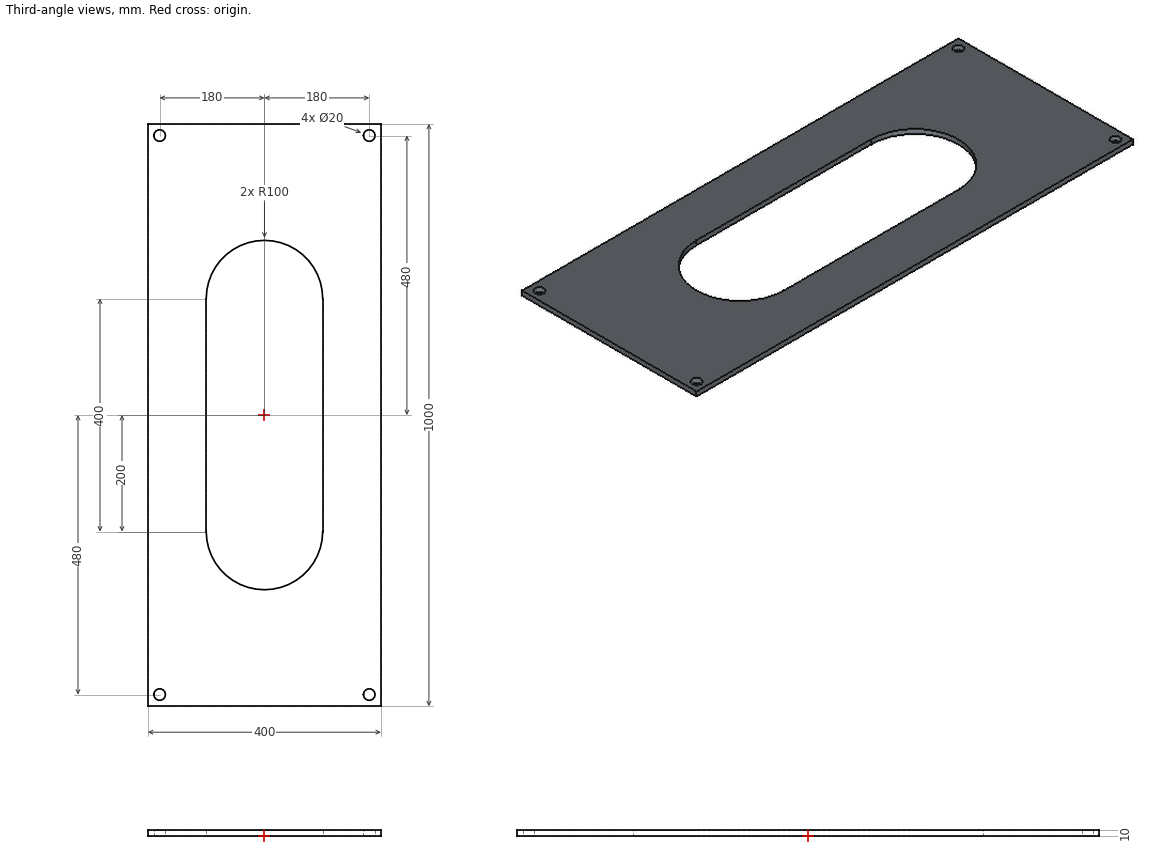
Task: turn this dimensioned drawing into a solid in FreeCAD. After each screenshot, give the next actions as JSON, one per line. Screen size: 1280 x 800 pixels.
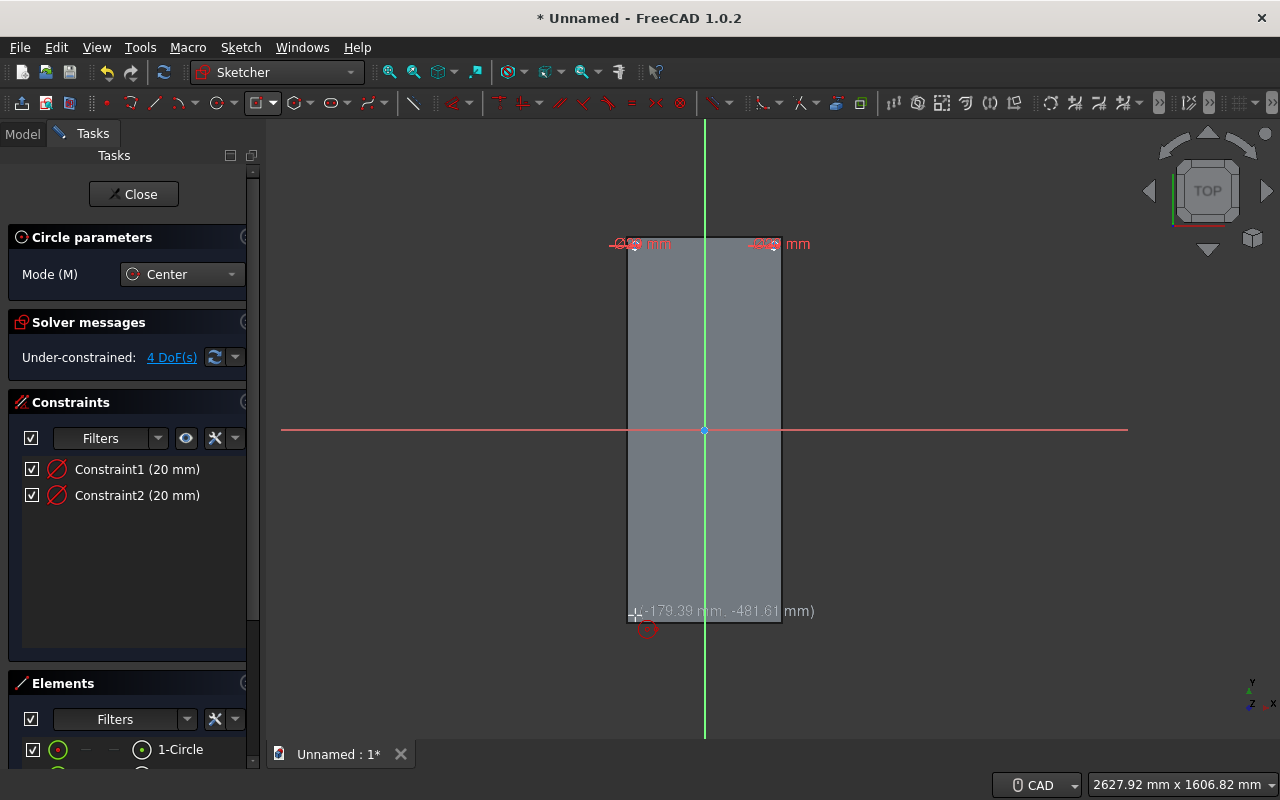
{"action": "left_click", "coordinate": [635, 615]}
{"action": "mouse_move", "coordinate": [638, 612]}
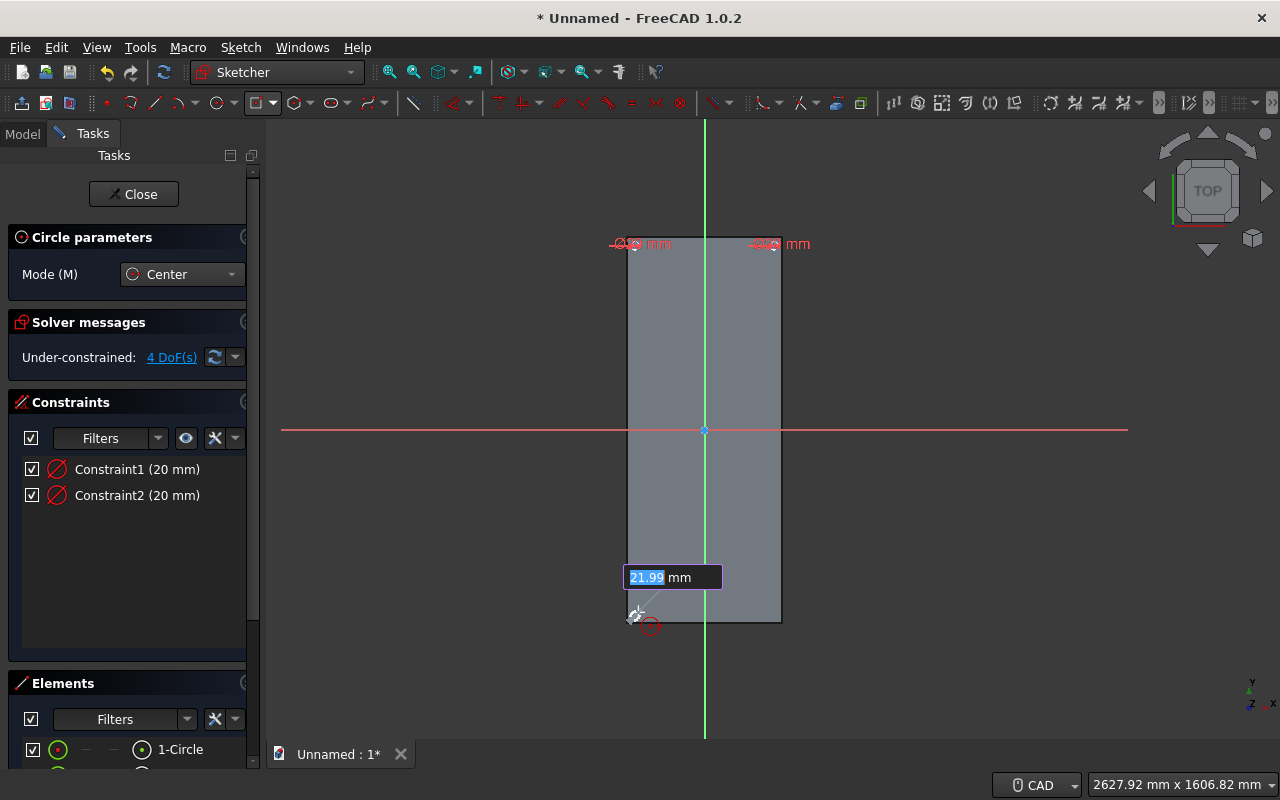
{"action": "type", "text": "20"}
{"action": "key", "text": "Return"}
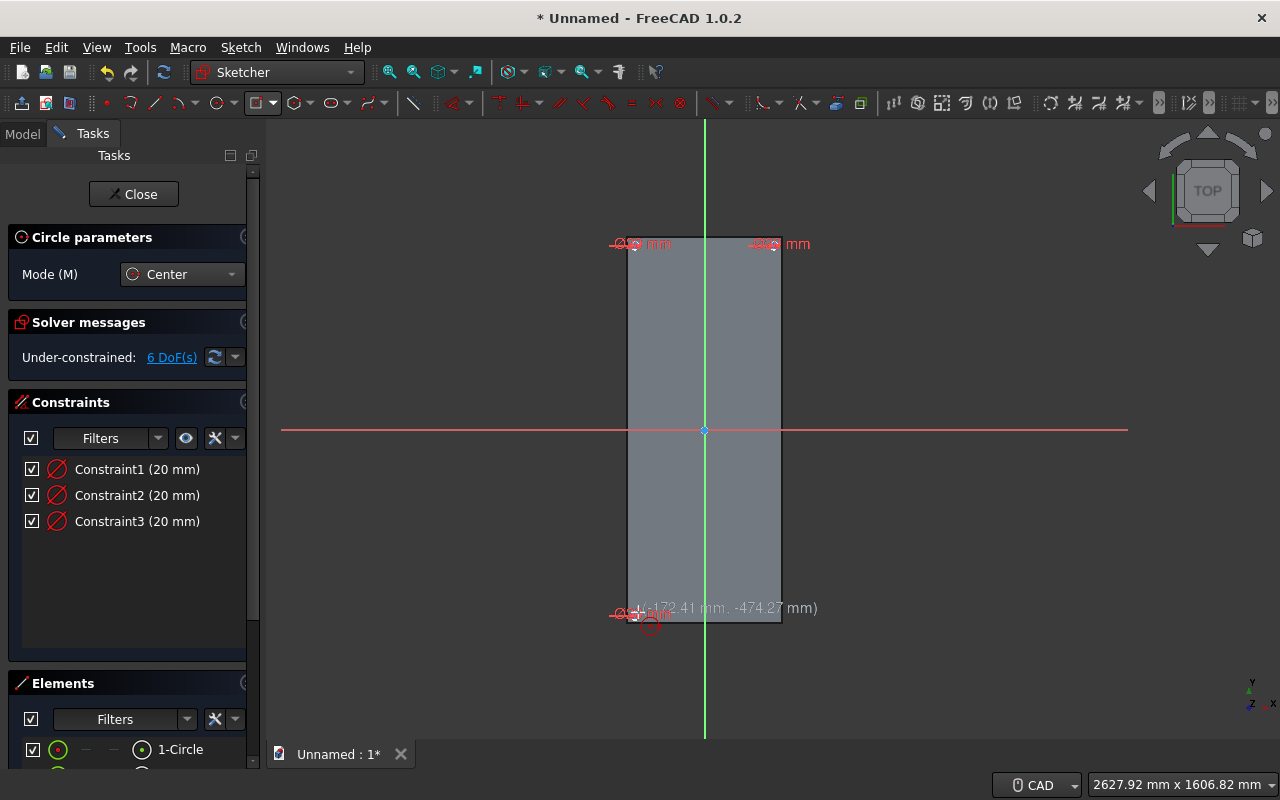
{"action": "scroll", "coordinate": [774, 615], "scroll_direction": "up", "scroll_amount": 9}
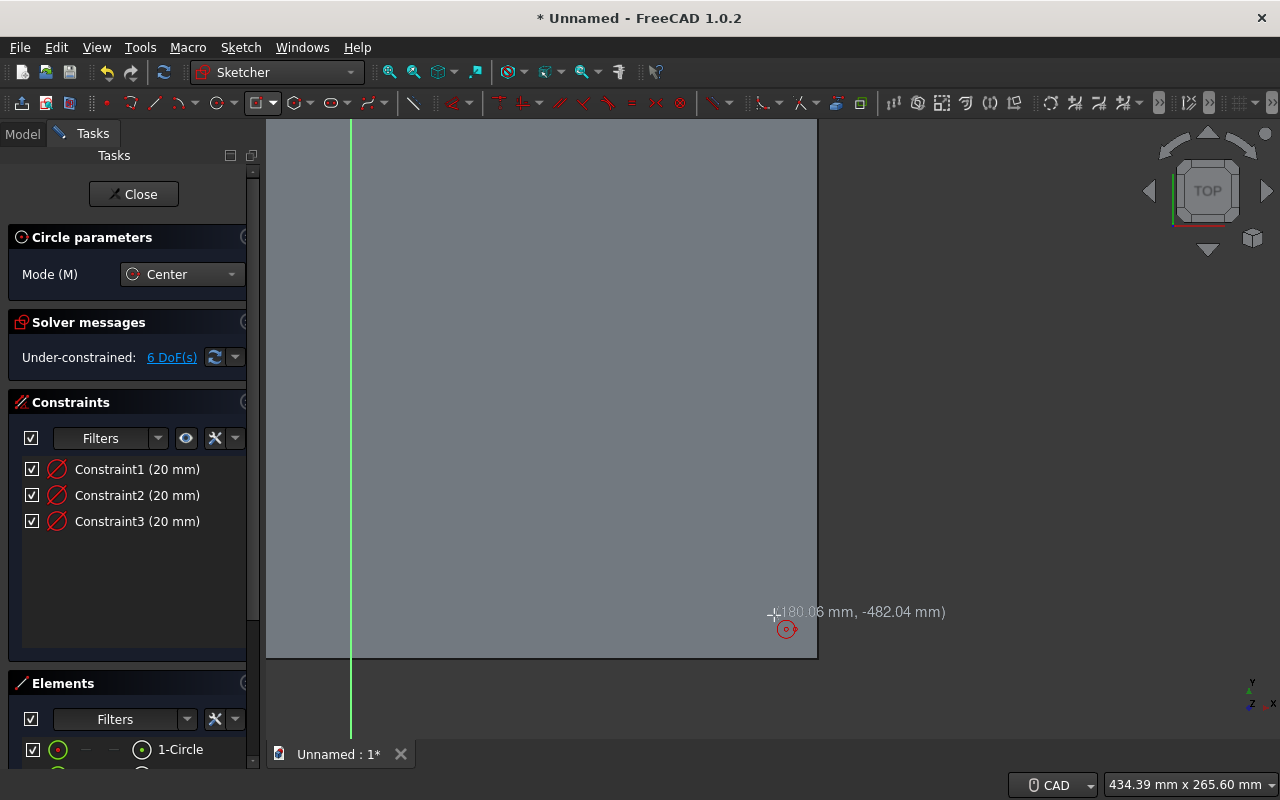
{"action": "scroll", "coordinate": [774, 615], "scroll_direction": "down", "scroll_amount": 9}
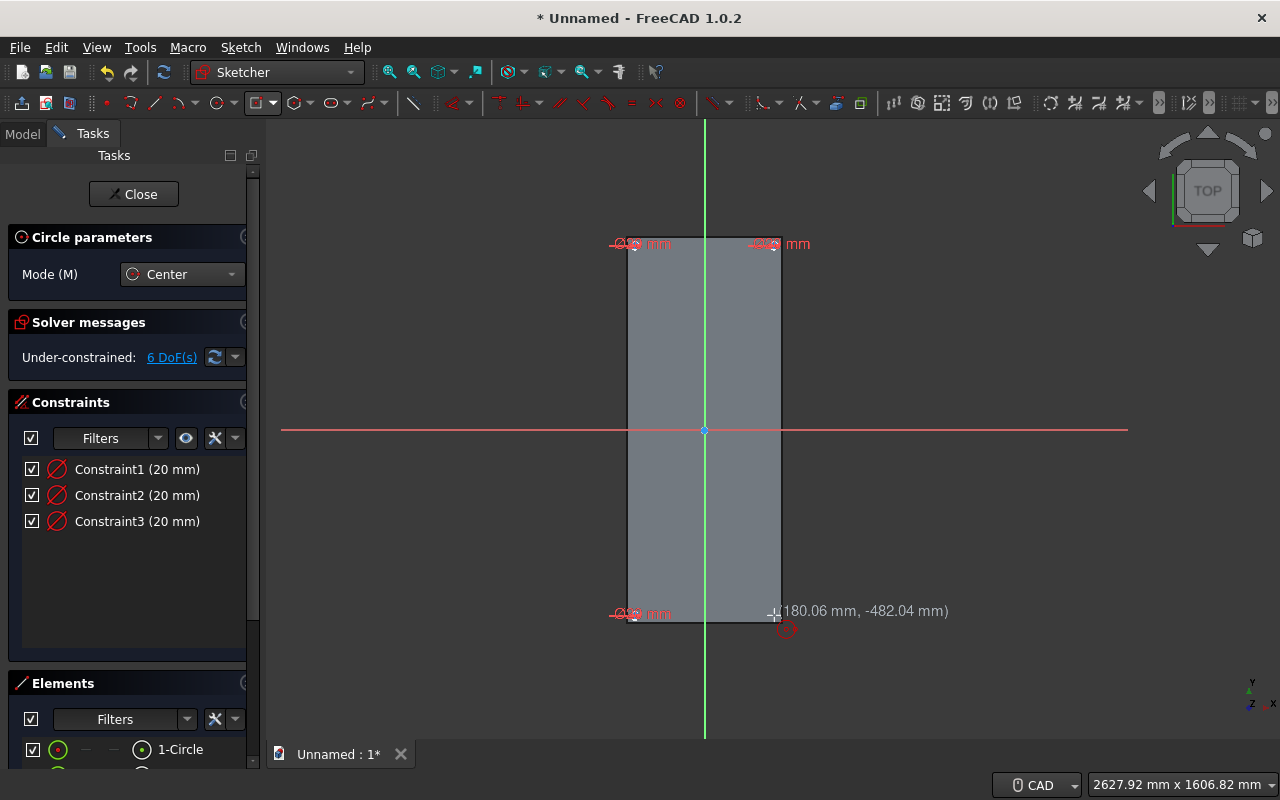
{"action": "left_click", "coordinate": [774, 615]}
{"action": "mouse_move", "coordinate": [777, 612]}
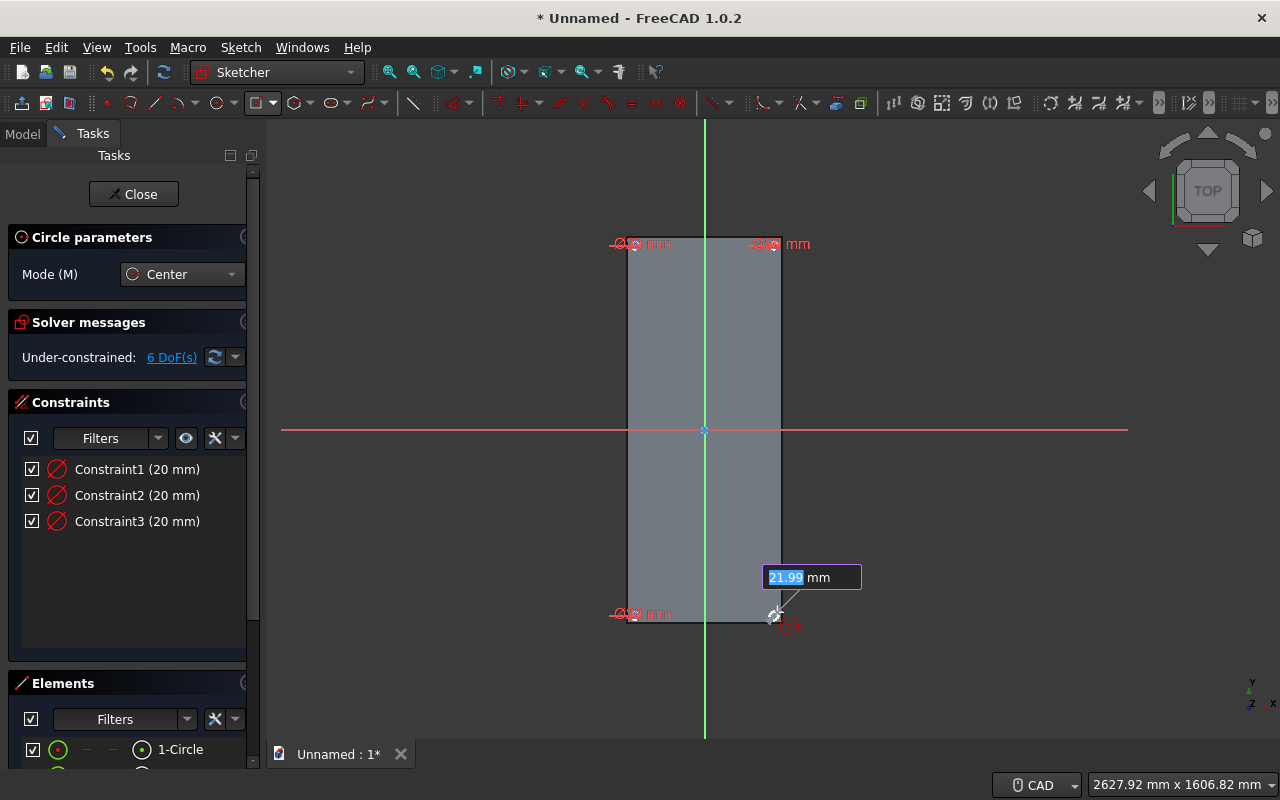
{"action": "type", "text": "20"}
{"action": "key", "text": "Return"}
{"action": "key", "text": "Escape"}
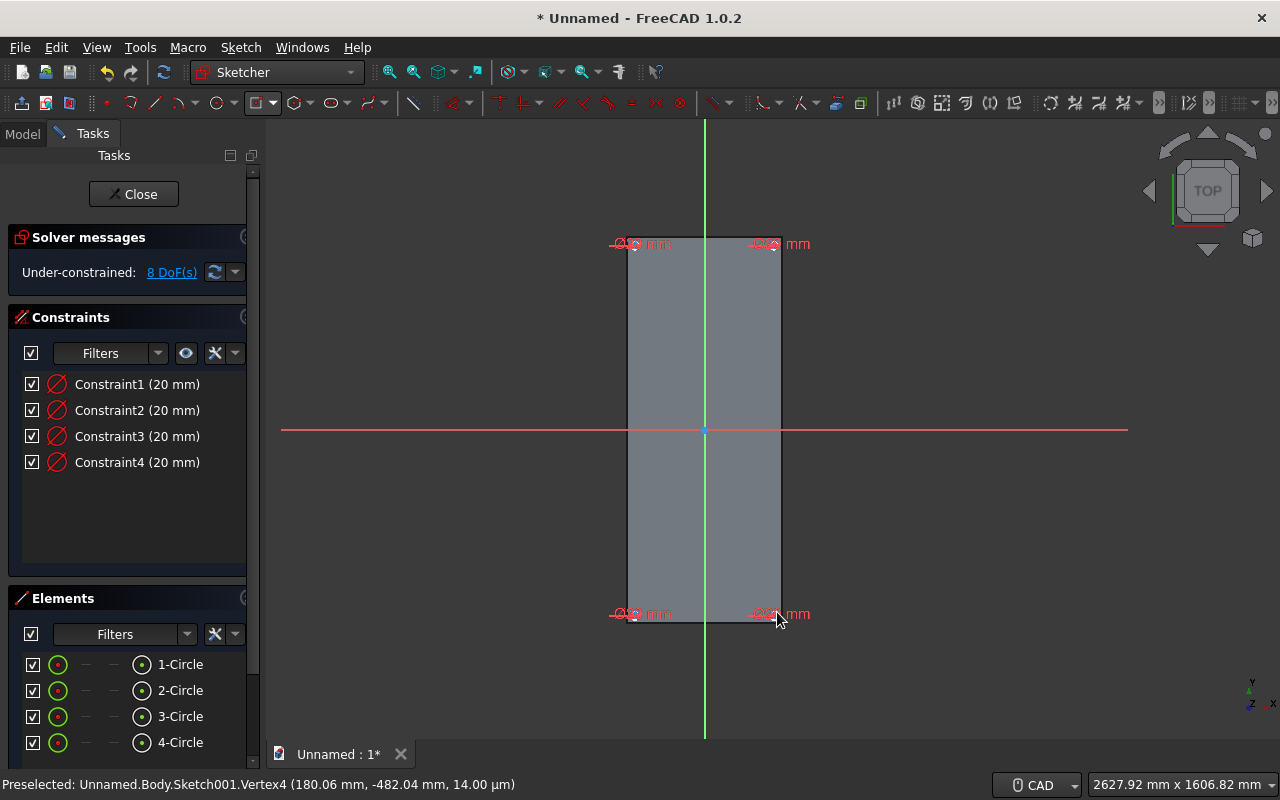
{"action": "left_click", "coordinate": [774, 246]}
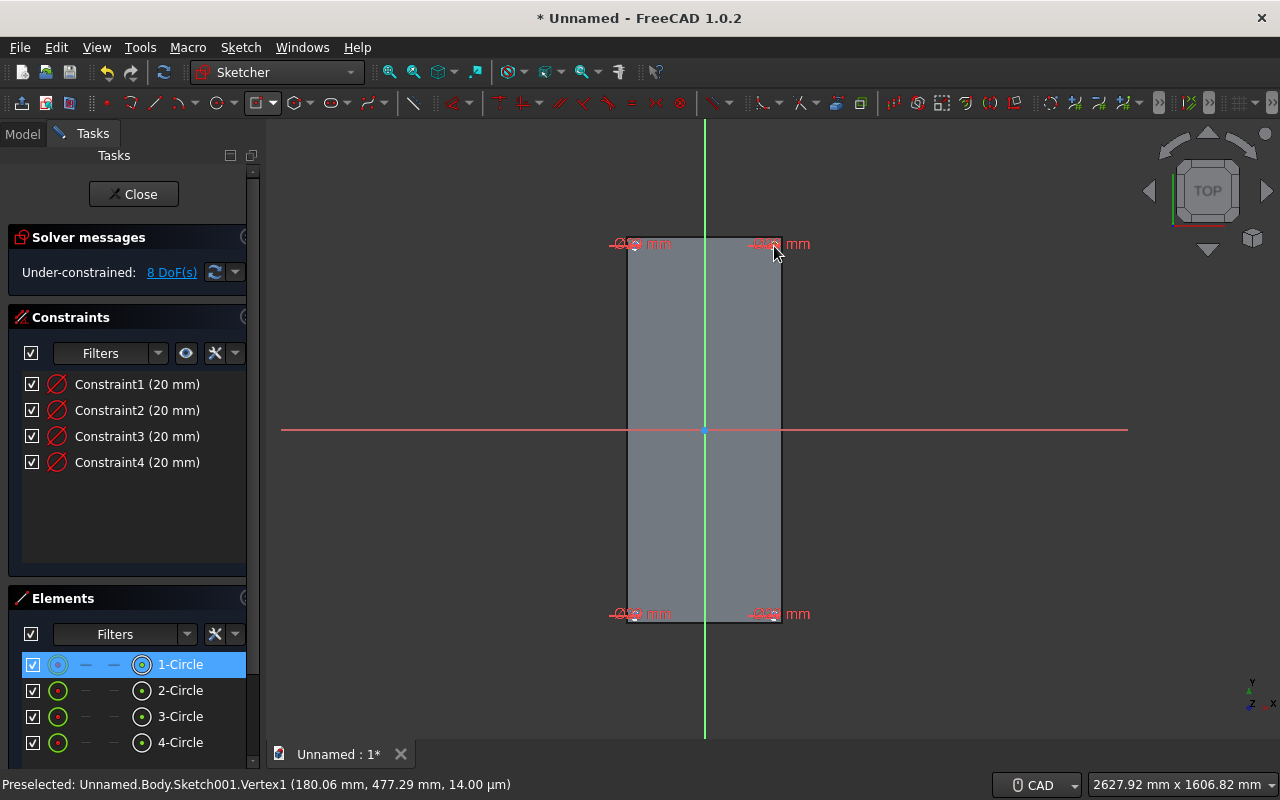
{"action": "left_click", "coordinate": [635, 246]}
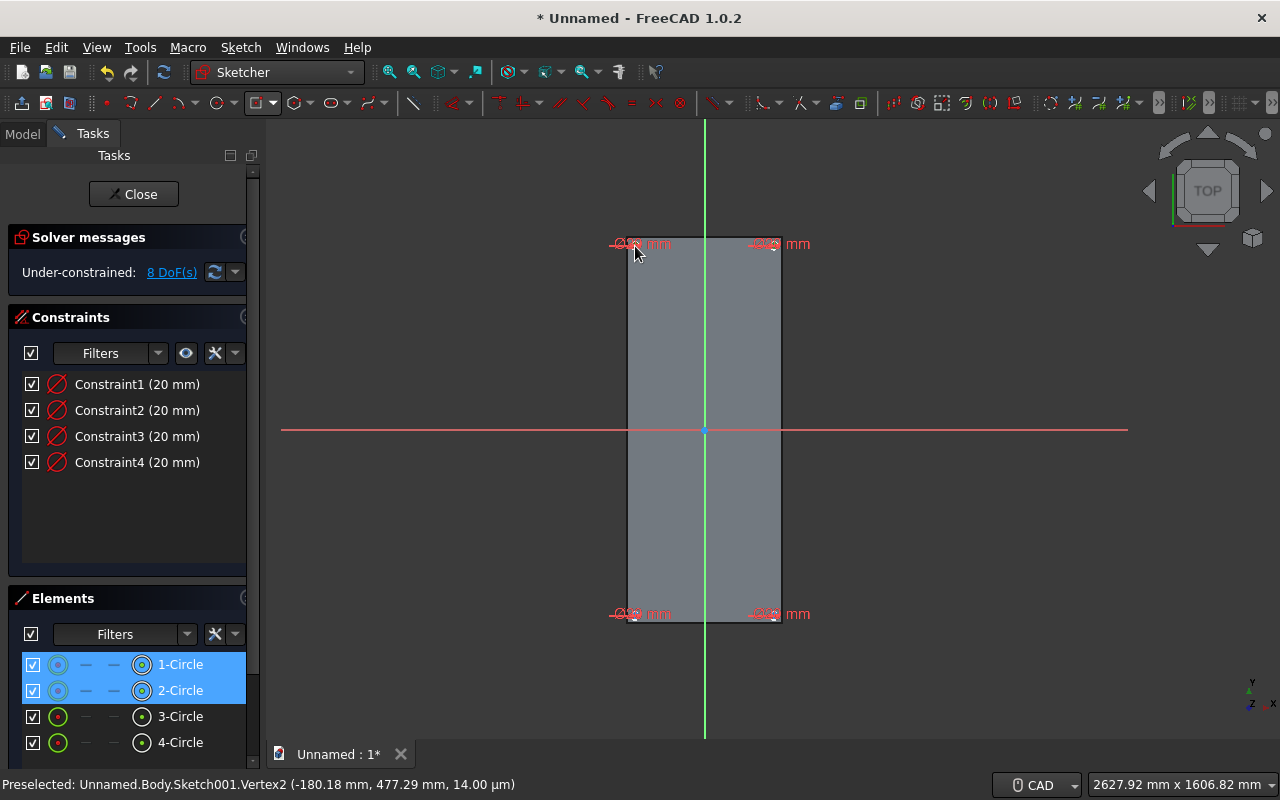
{"action": "key", "text": "h"}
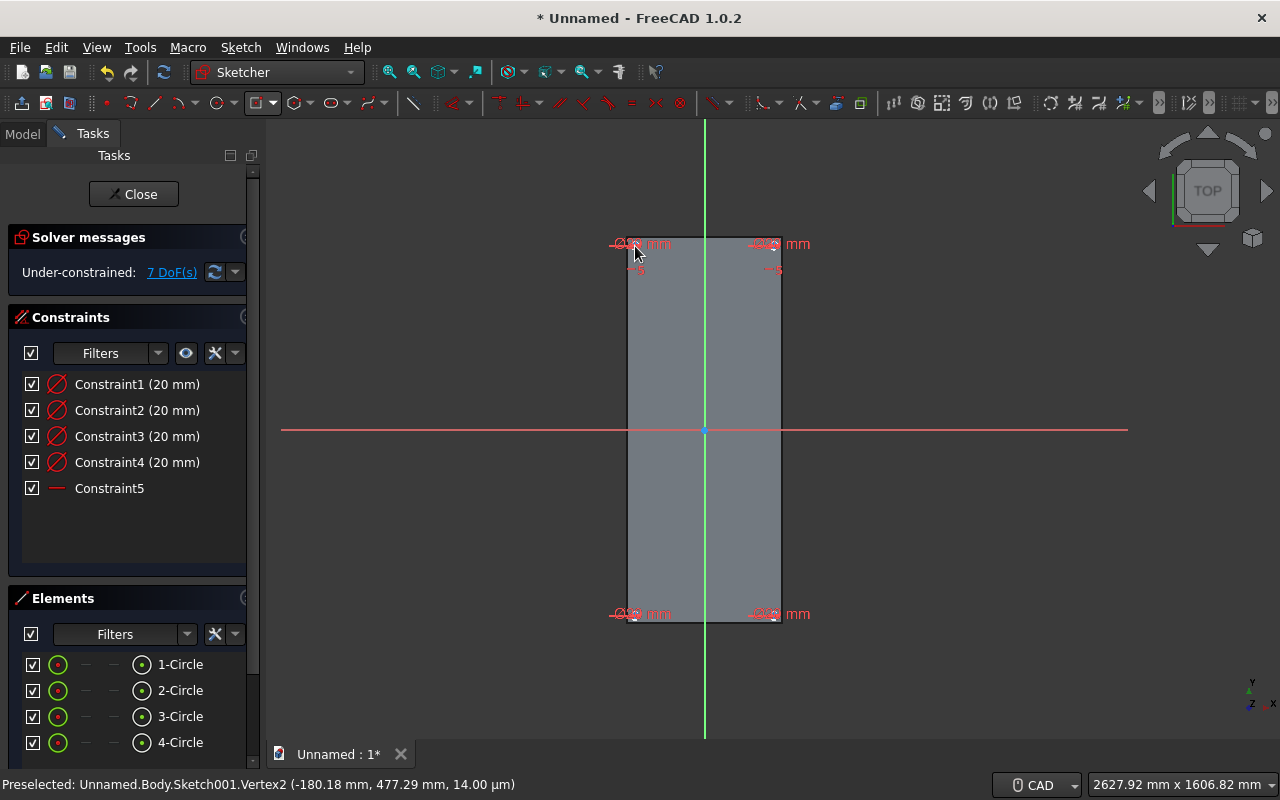
{"action": "left_click", "coordinate": [635, 246]}